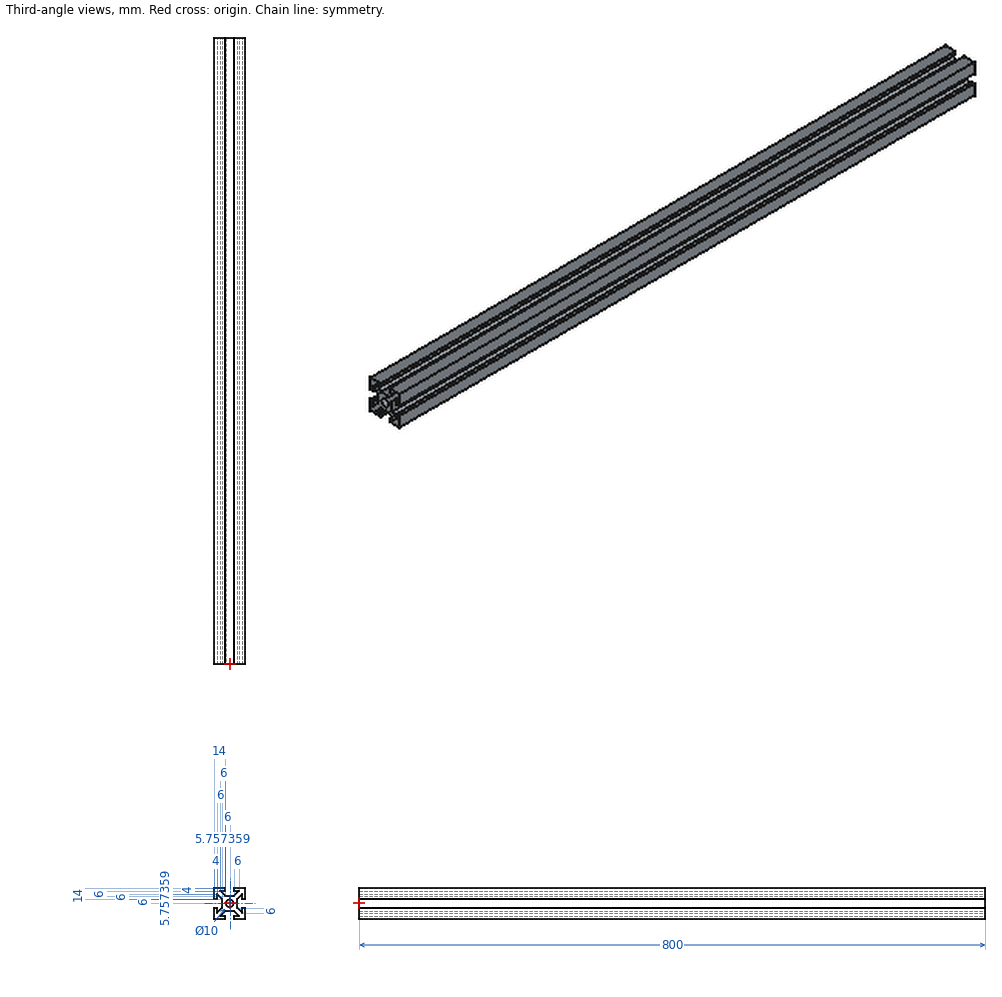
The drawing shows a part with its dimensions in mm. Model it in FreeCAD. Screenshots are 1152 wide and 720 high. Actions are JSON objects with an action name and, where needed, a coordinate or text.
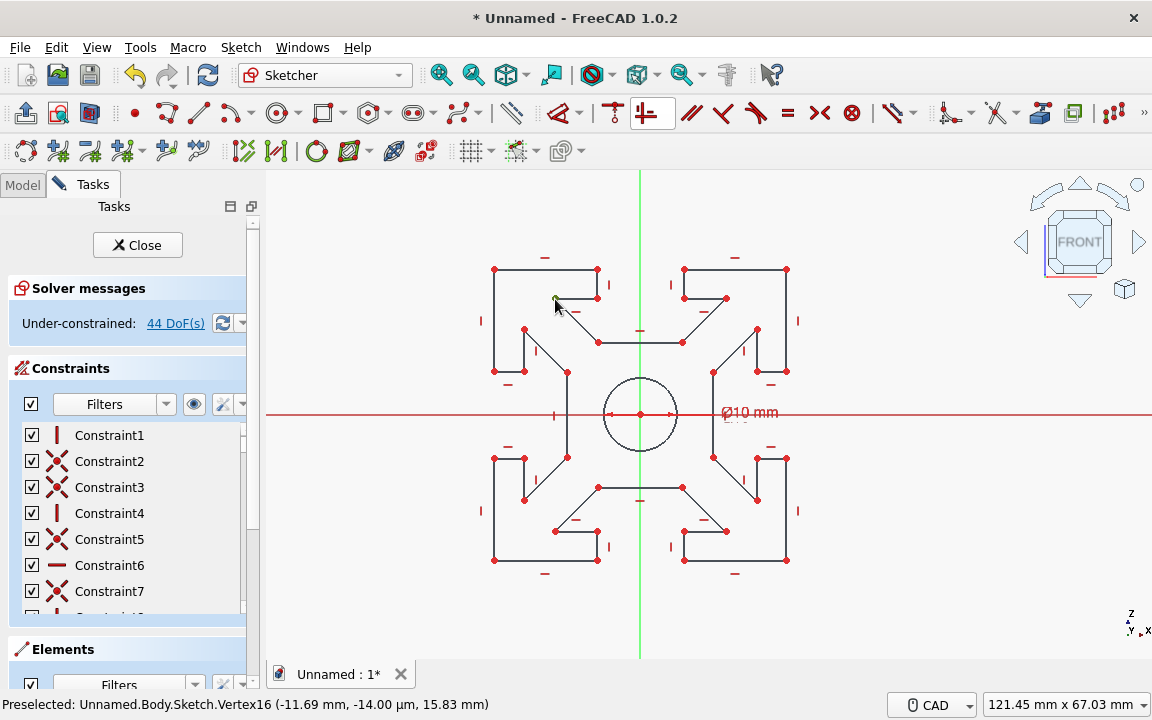
{"action": "left_click", "coordinate": [726, 299]}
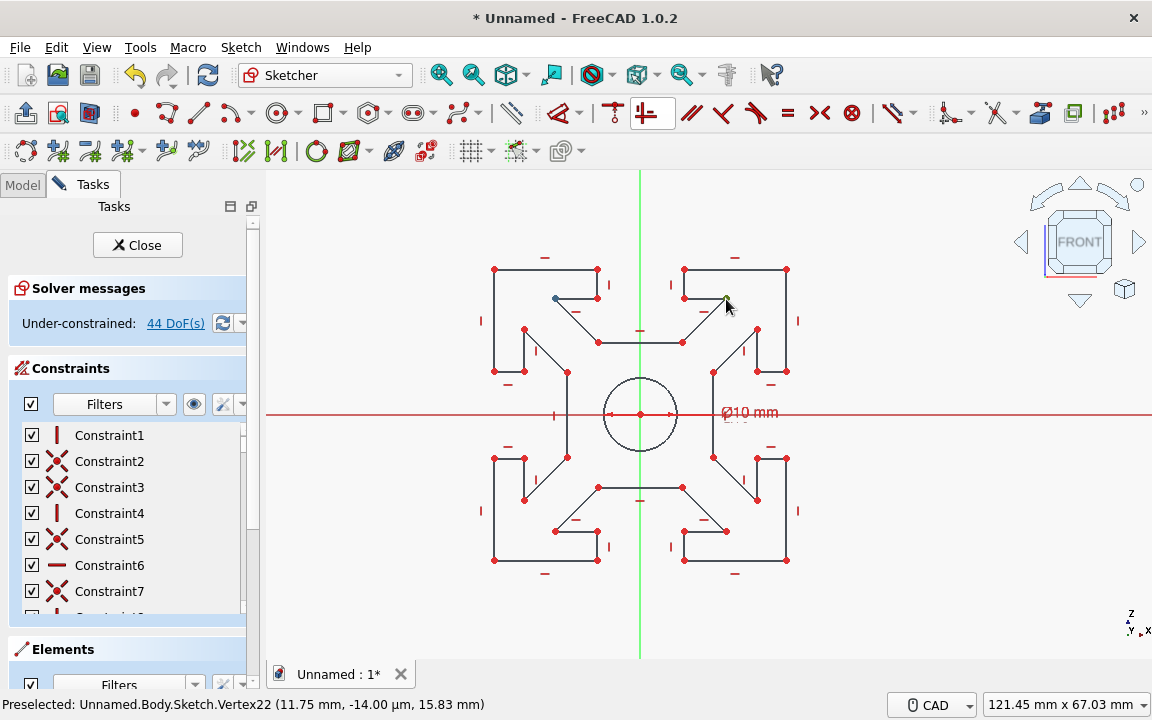
{"action": "left_click", "coordinate": [640, 600]}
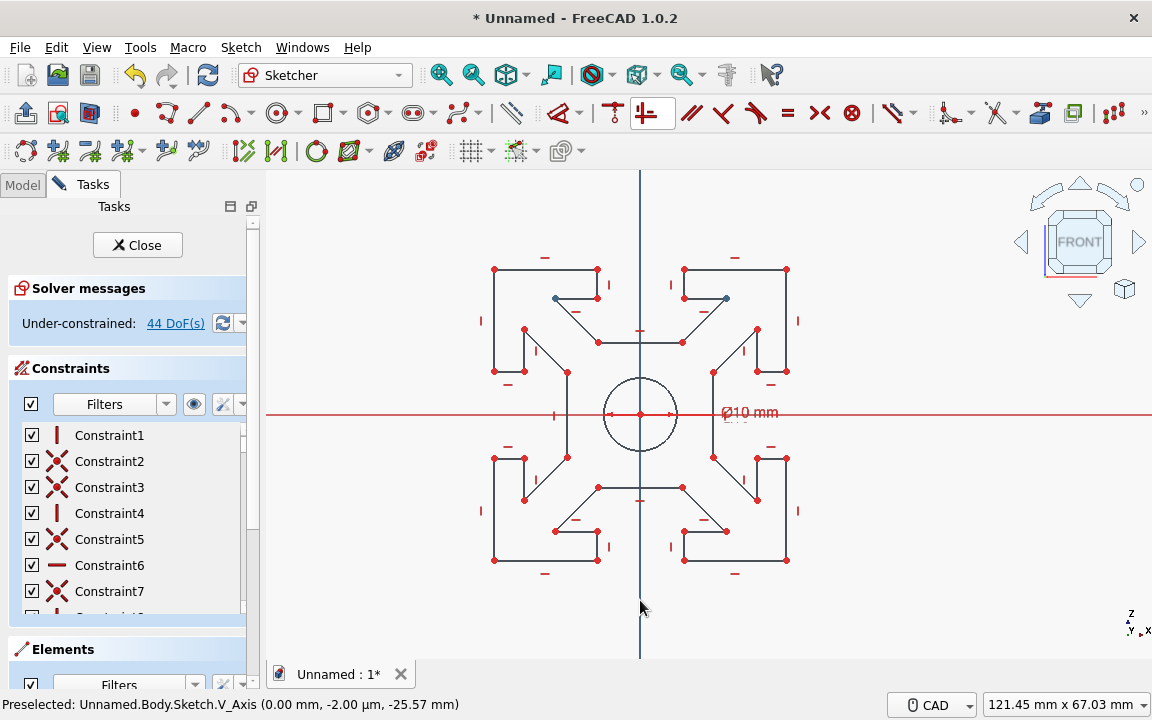
{"action": "key", "text": "s"}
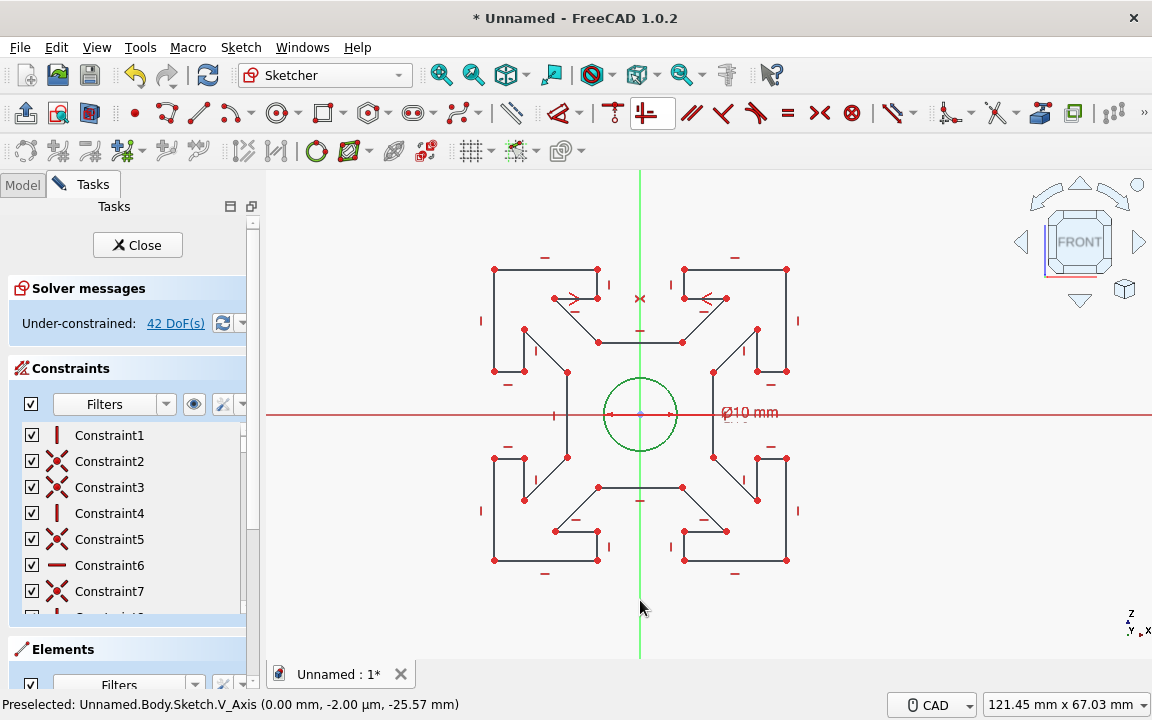
{"action": "left_click", "coordinate": [597, 270]}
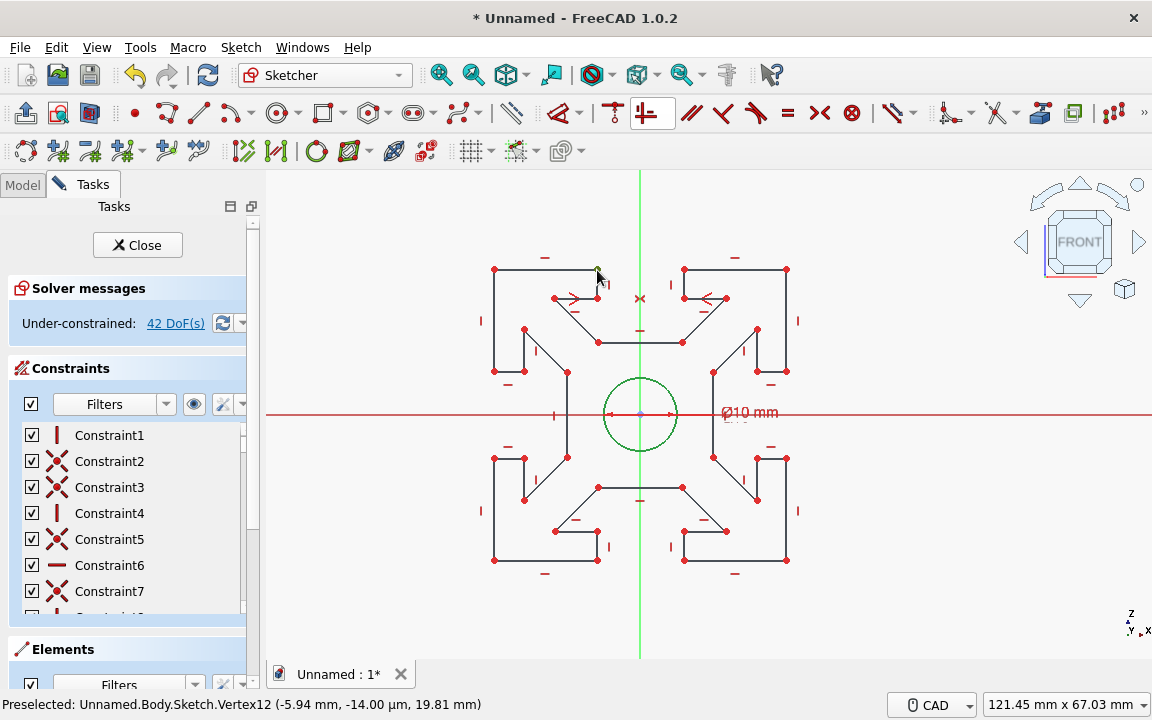
{"action": "left_click", "coordinate": [684, 270]}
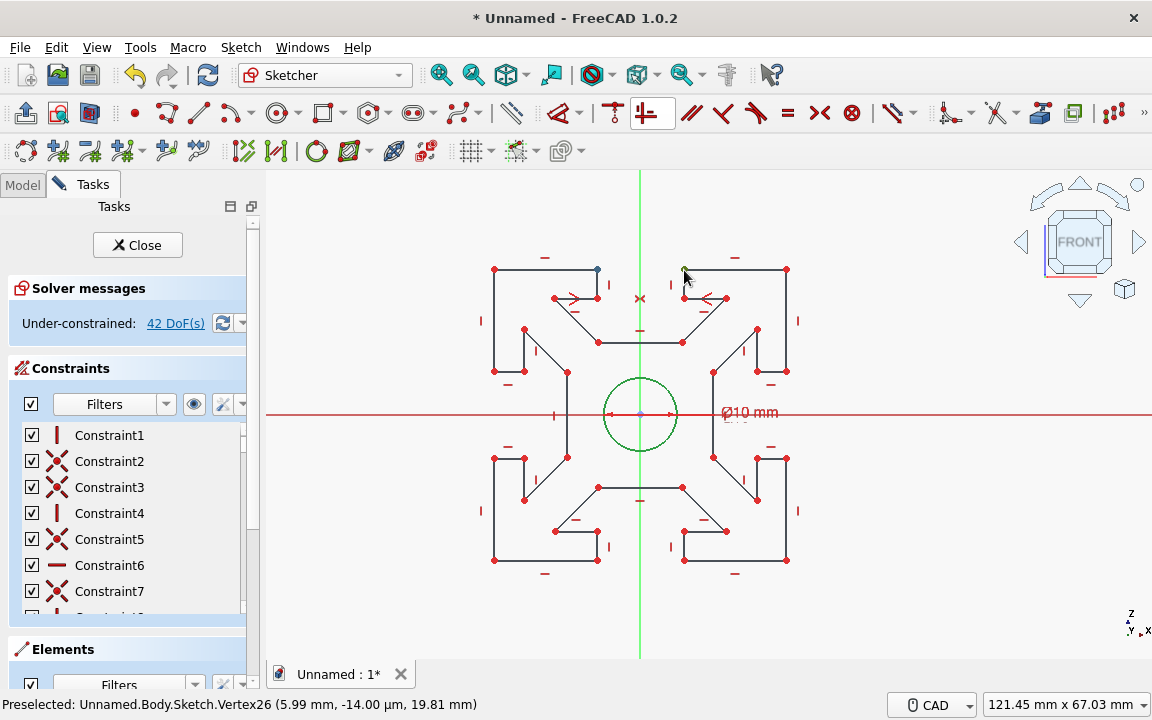
{"action": "left_click", "coordinate": [640, 600]}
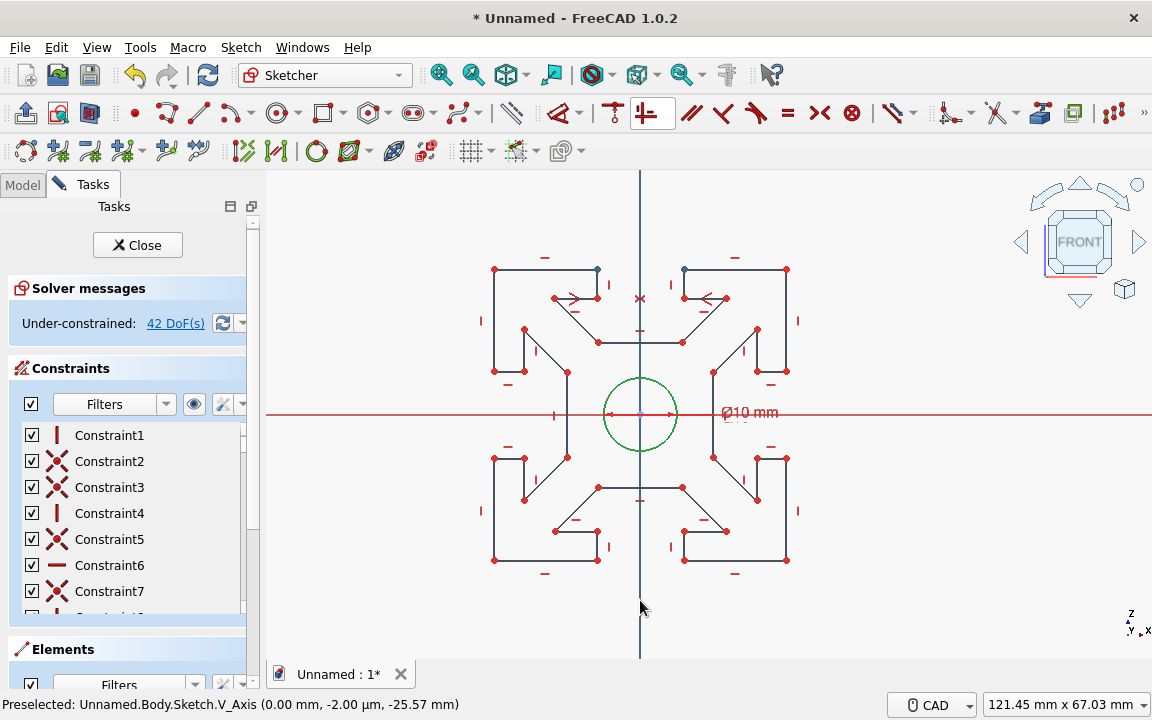
{"action": "left_click", "coordinate": [820, 114]}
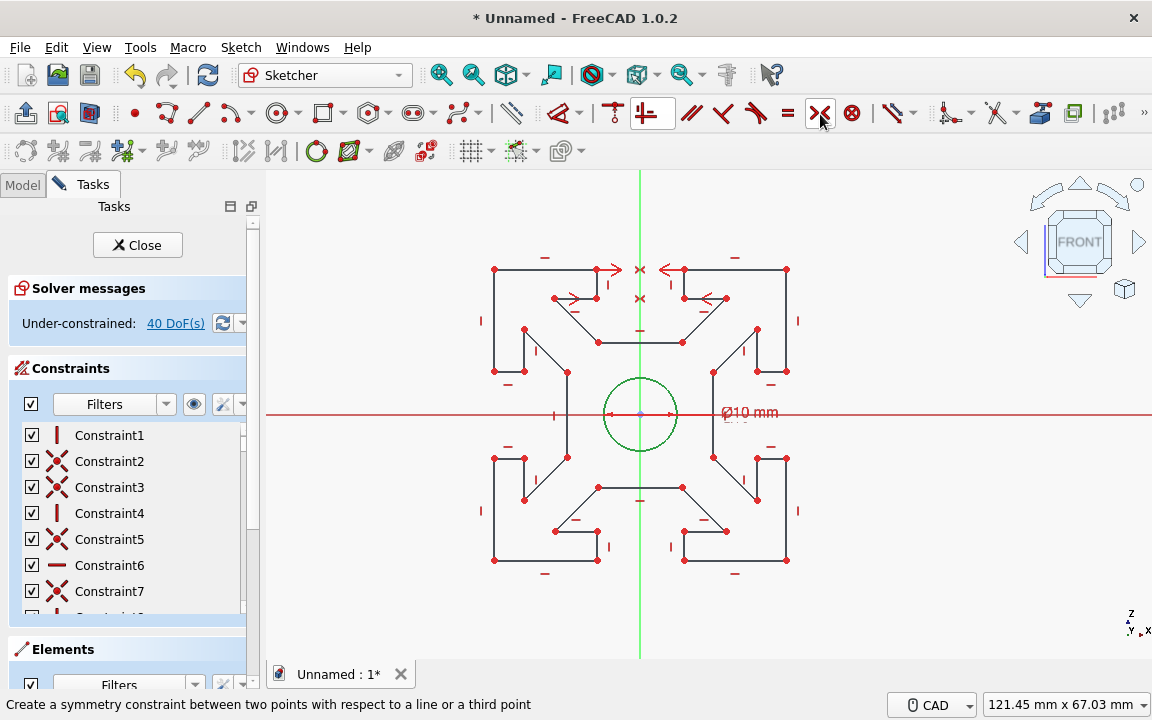
{"action": "left_click", "coordinate": [494, 372]}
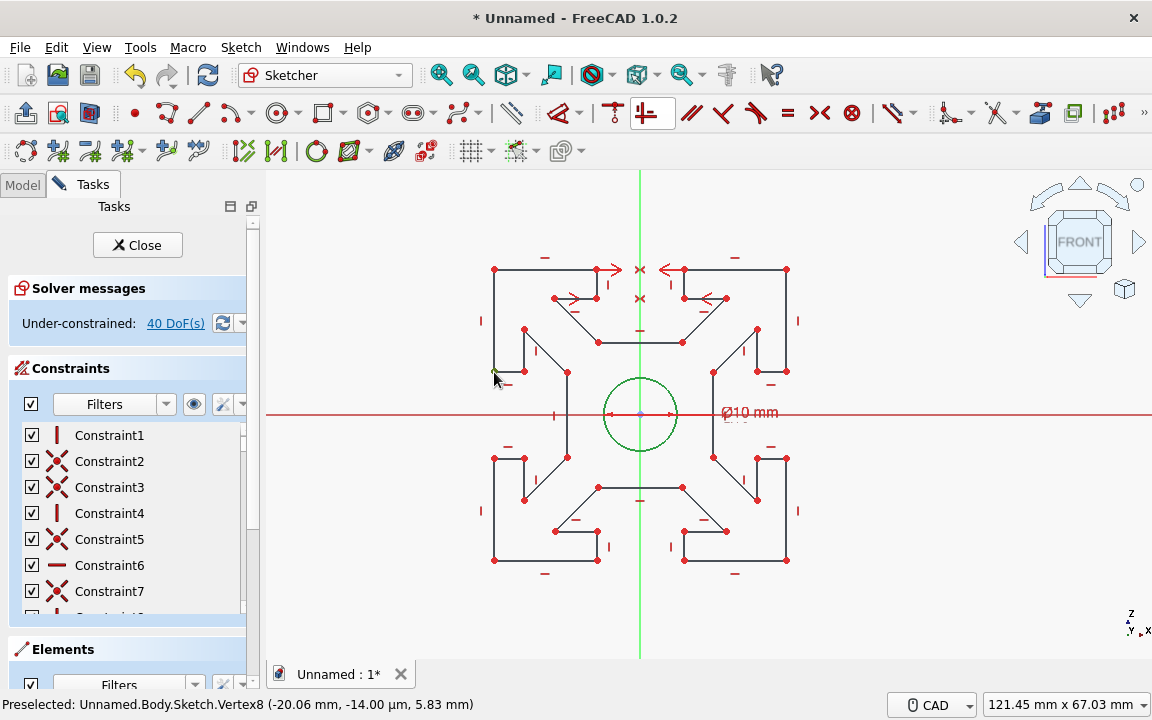
{"action": "left_click", "coordinate": [786, 372]}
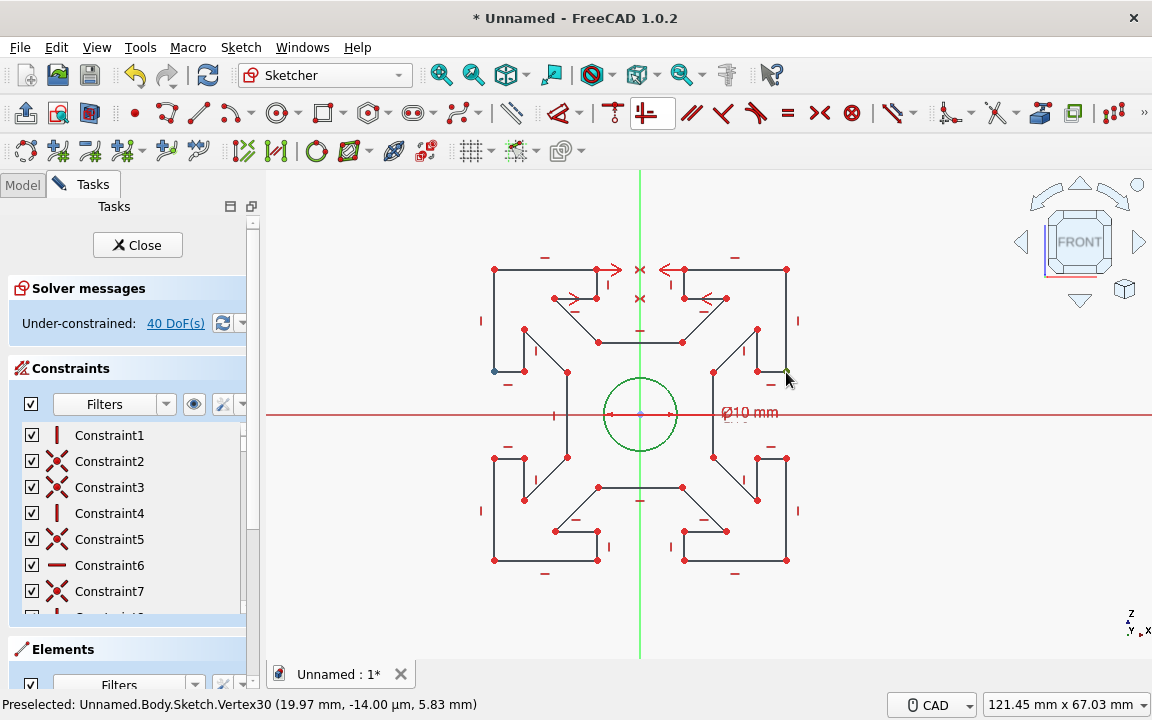
{"action": "left_click", "coordinate": [640, 600]}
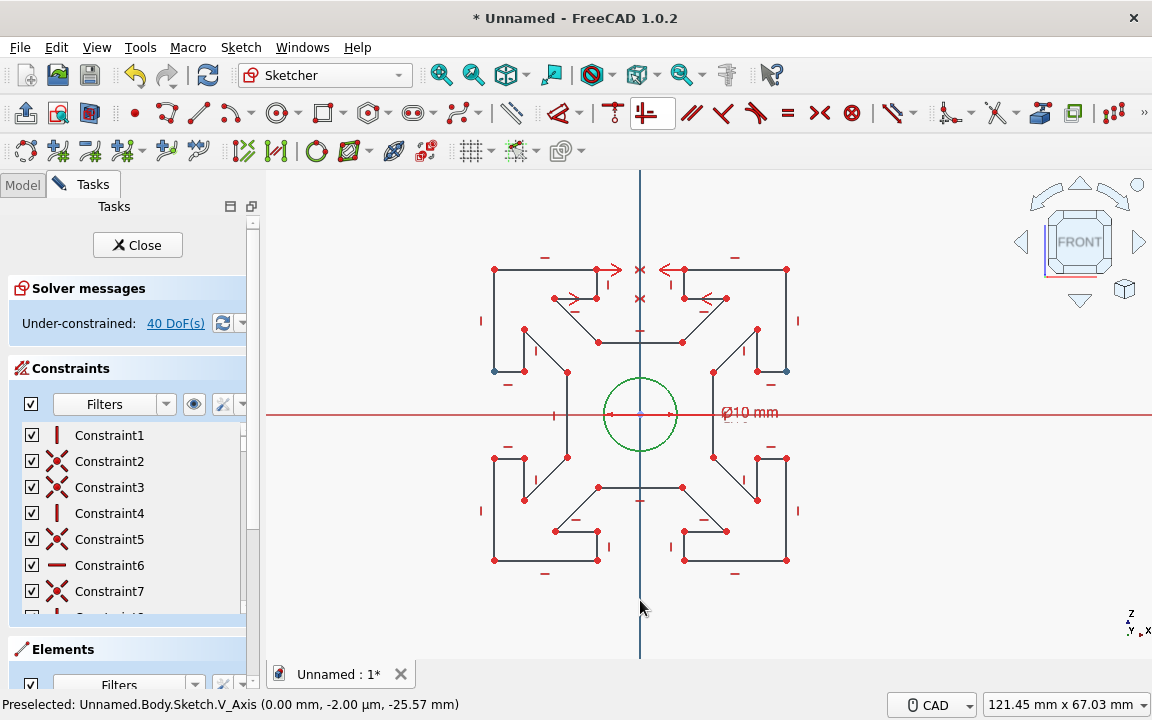
{"action": "key", "text": "s"}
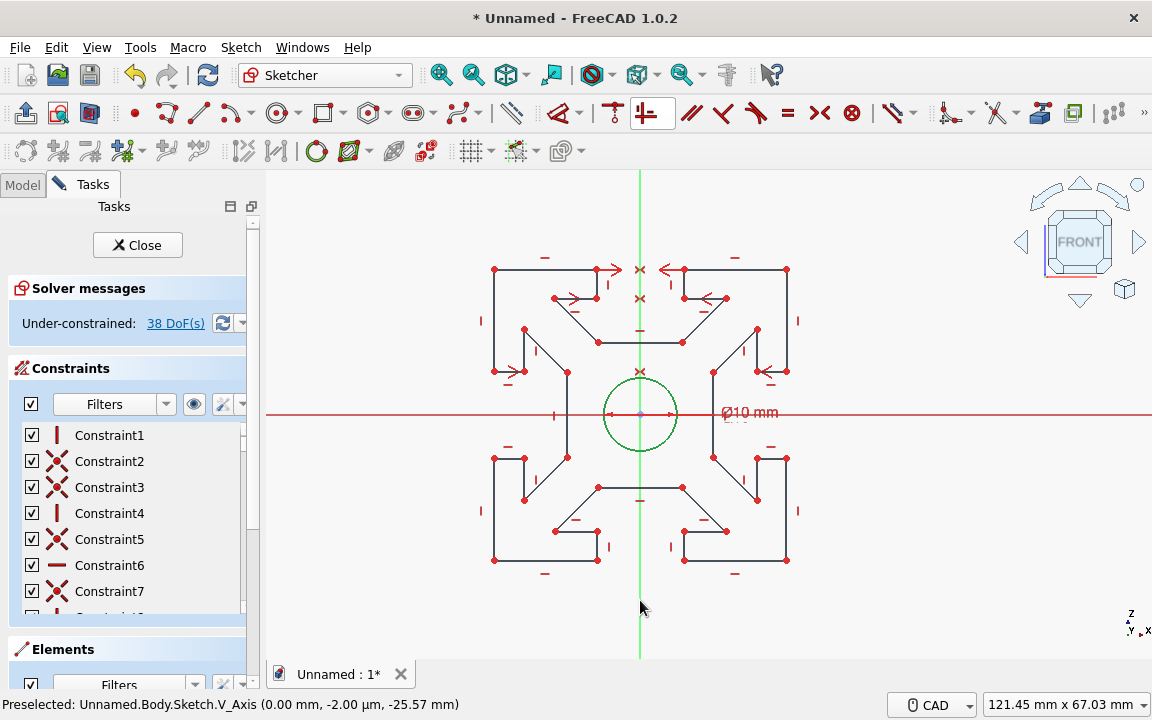
{"action": "left_click", "coordinate": [524, 330]}